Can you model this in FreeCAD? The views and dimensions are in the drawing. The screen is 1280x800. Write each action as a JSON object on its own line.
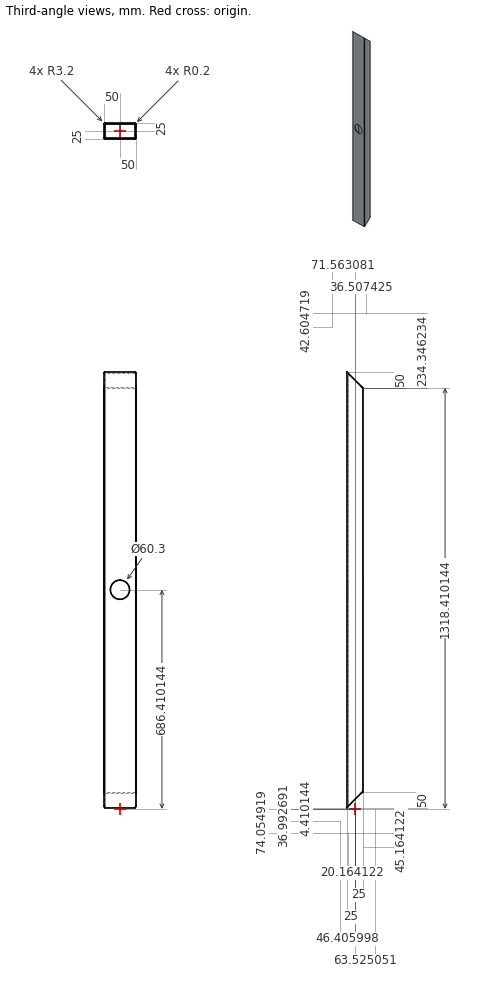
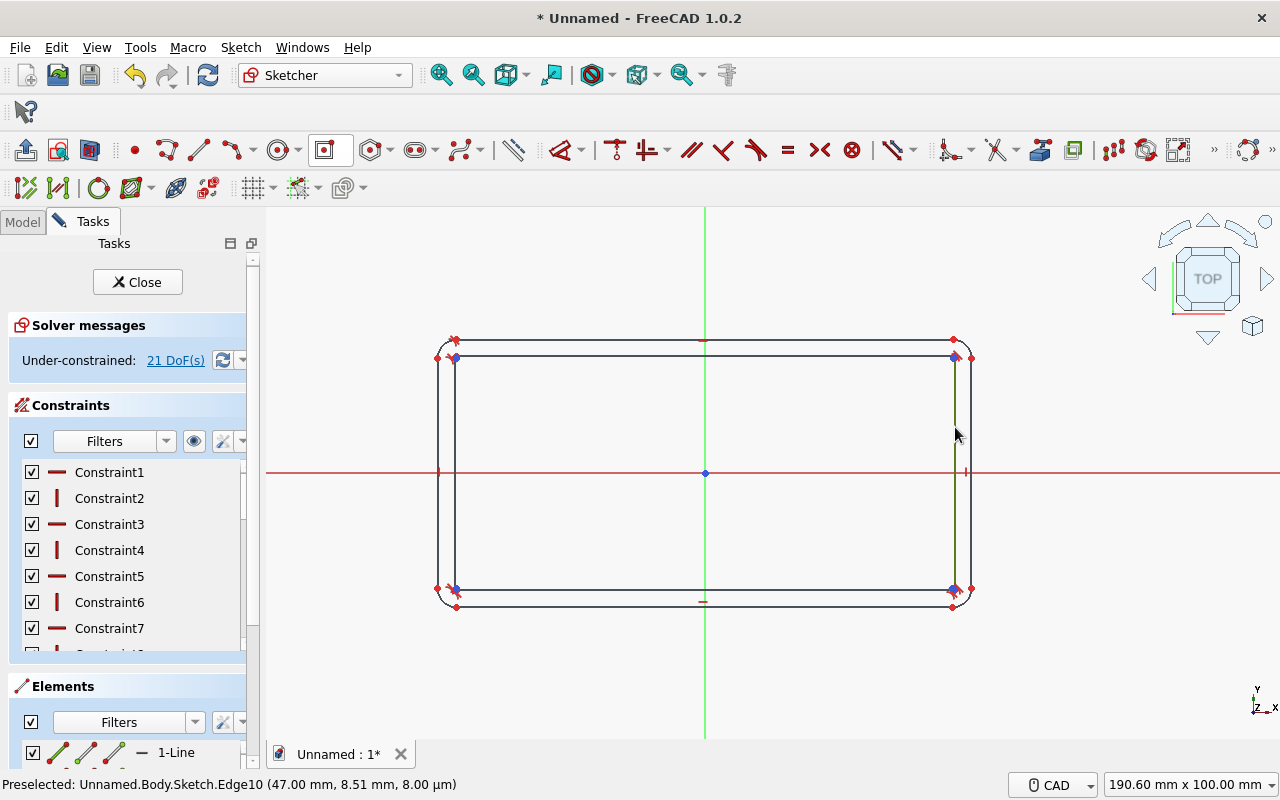
{"action": "scroll", "coordinate": [955, 590], "scroll_direction": "up", "scroll_amount": 14}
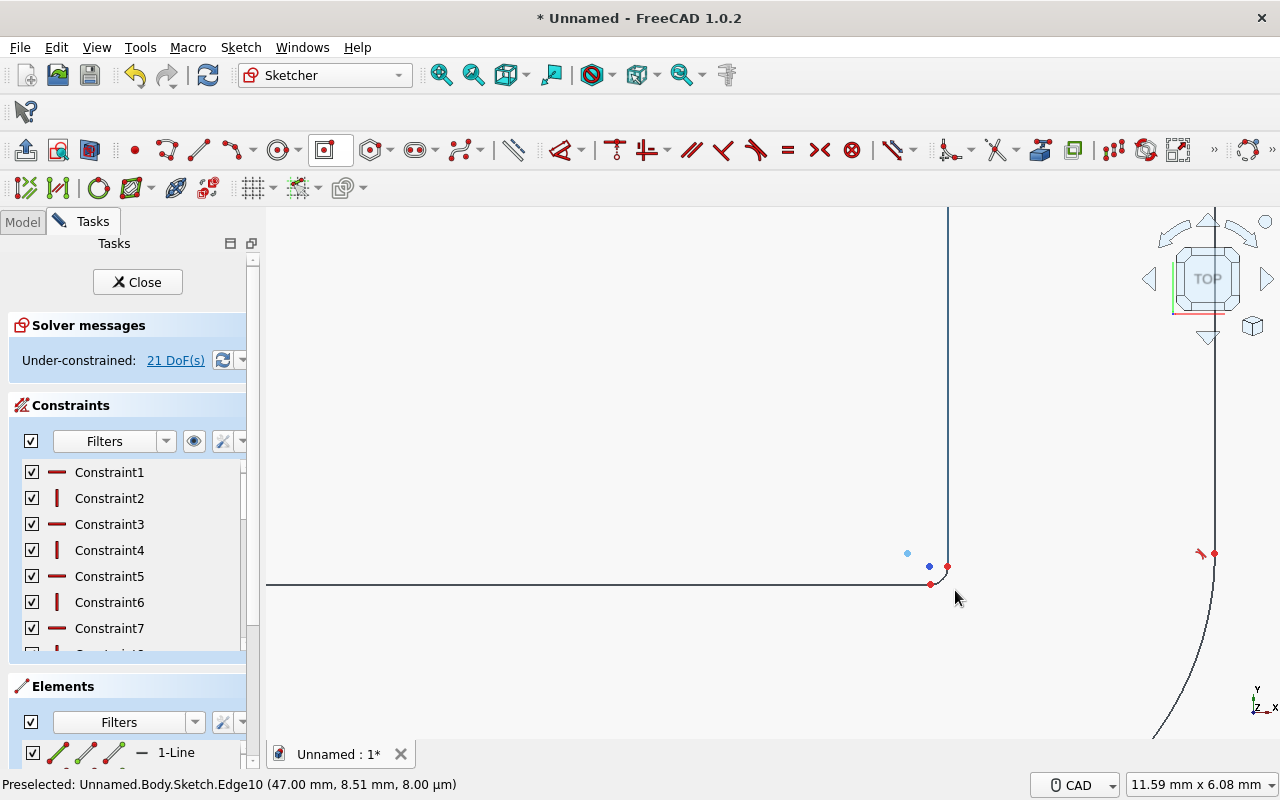
{"action": "left_click", "coordinate": [943, 579]}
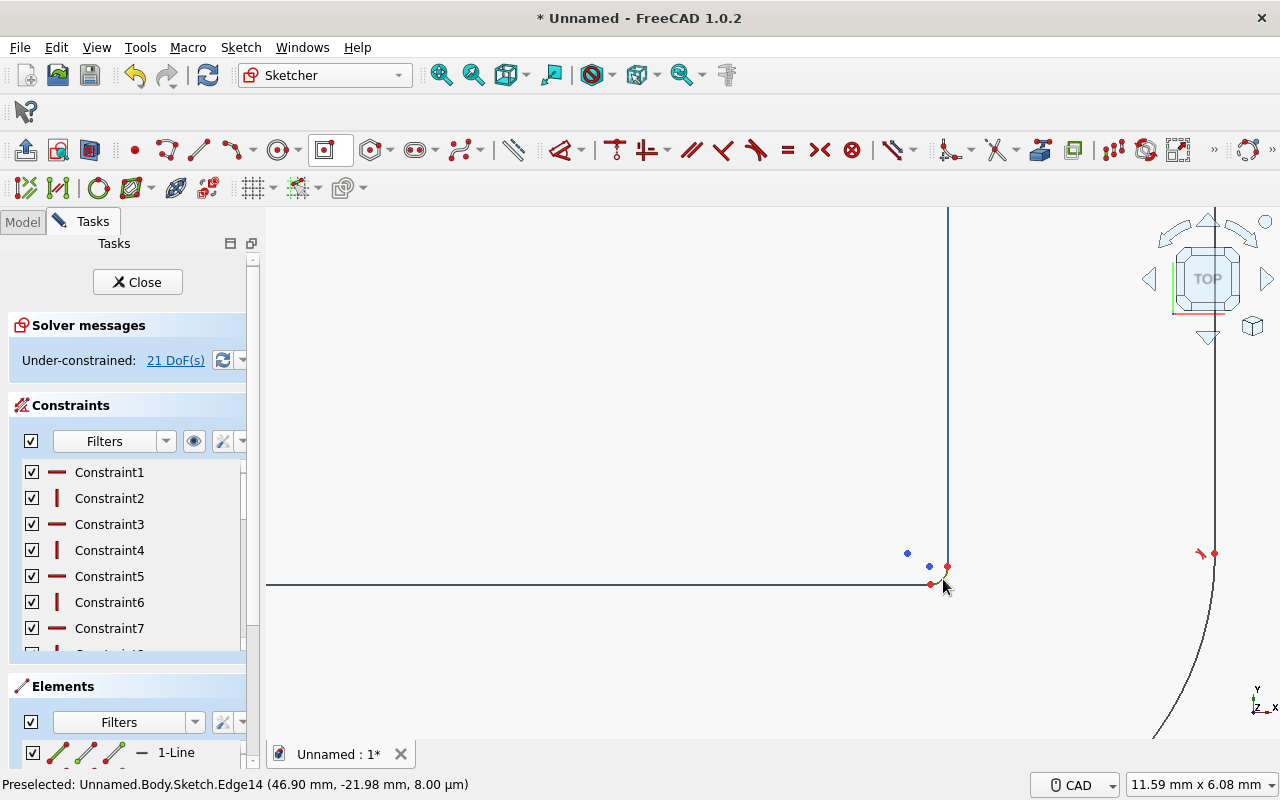
{"action": "key", "text": "t"}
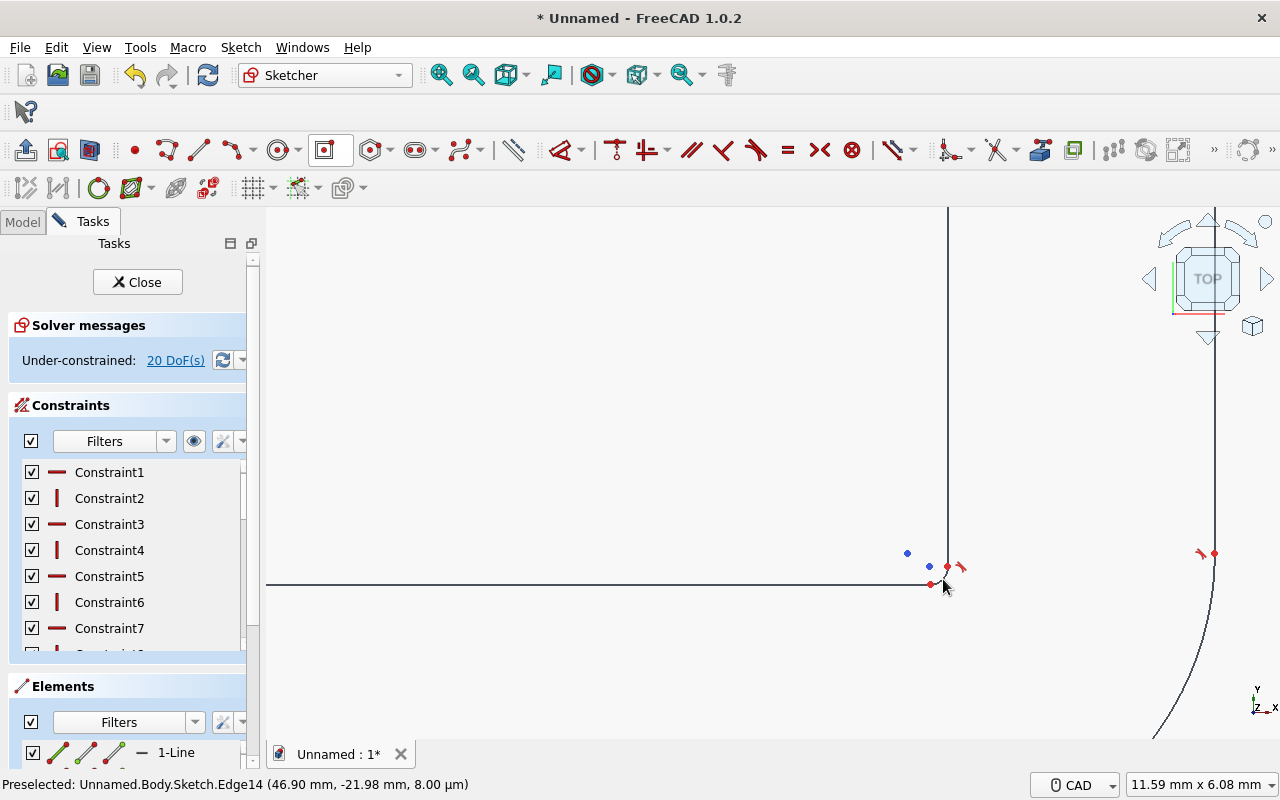
{"action": "scroll", "coordinate": [955, 590], "scroll_direction": "down", "scroll_amount": 14}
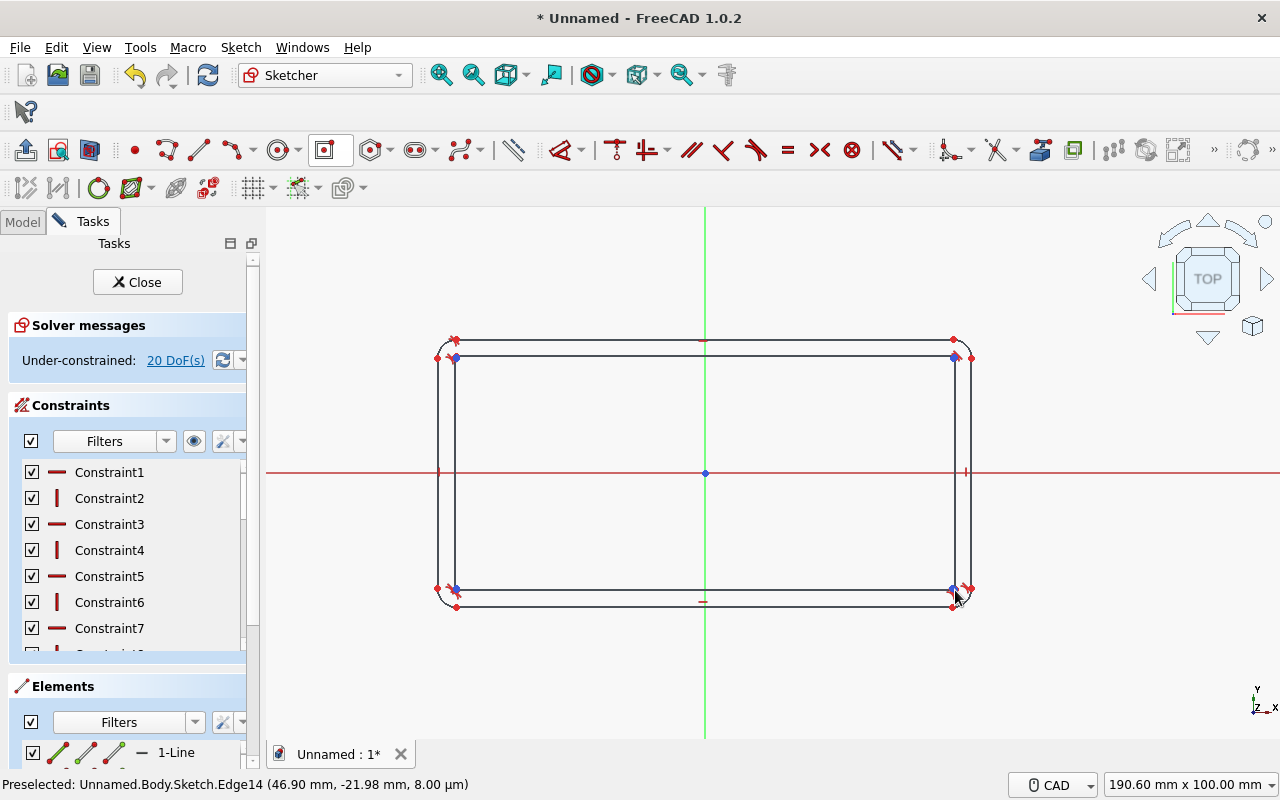
{"action": "left_click", "coordinate": [805, 590]}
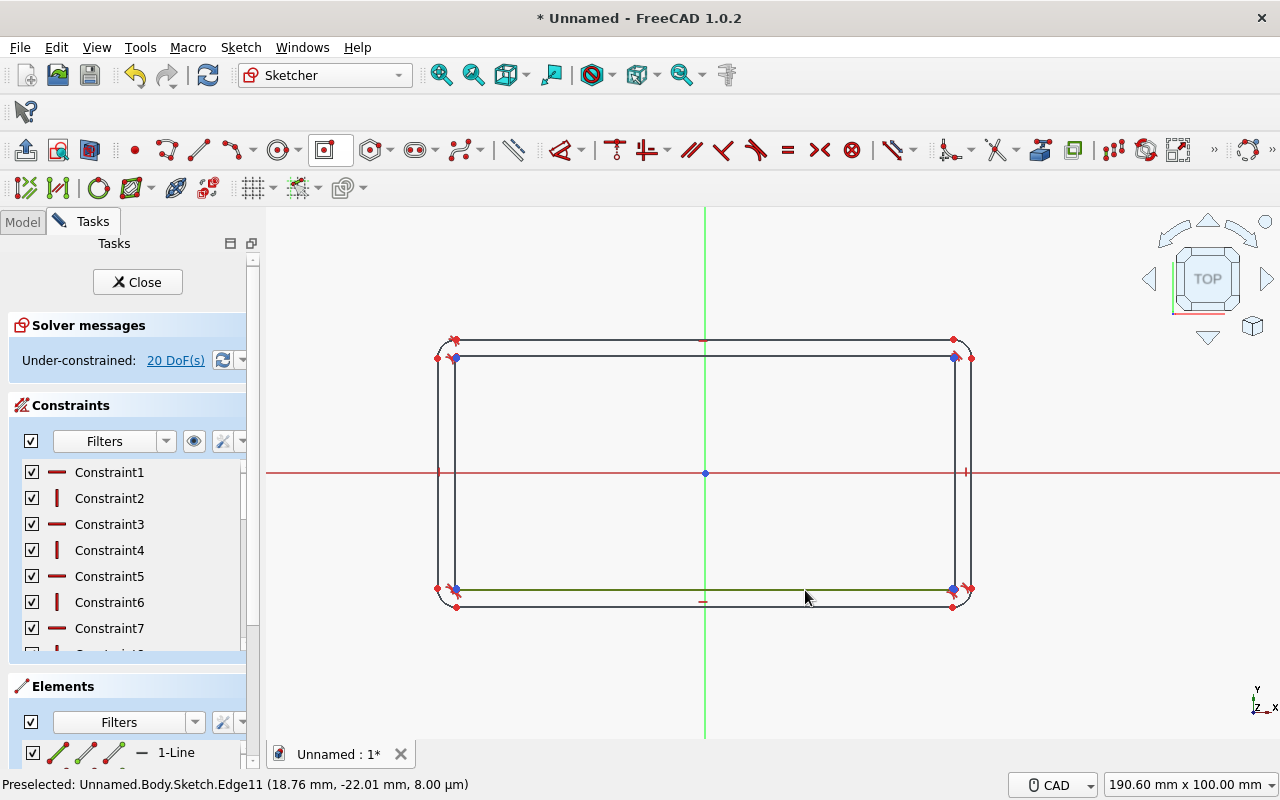
{"action": "scroll", "coordinate": [955, 590], "scroll_direction": "up", "scroll_amount": 14}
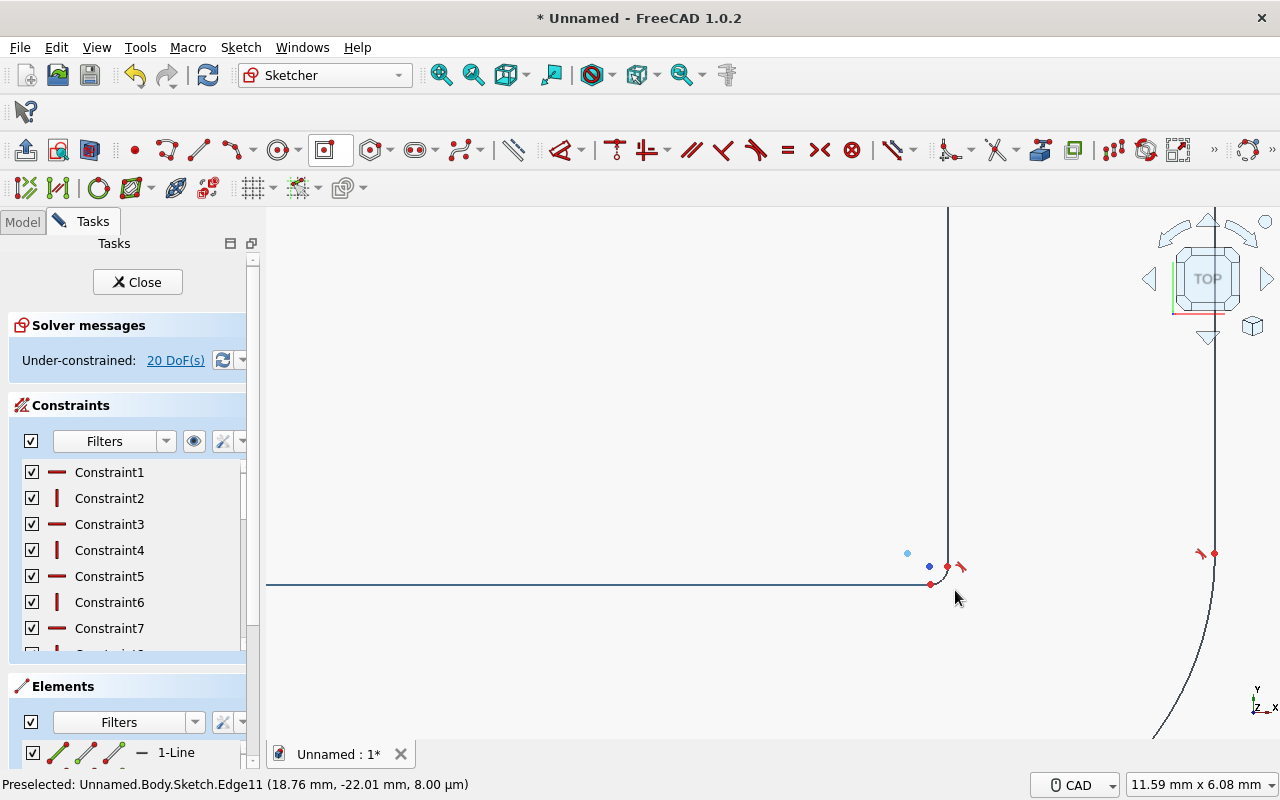
{"action": "left_click", "coordinate": [943, 579]}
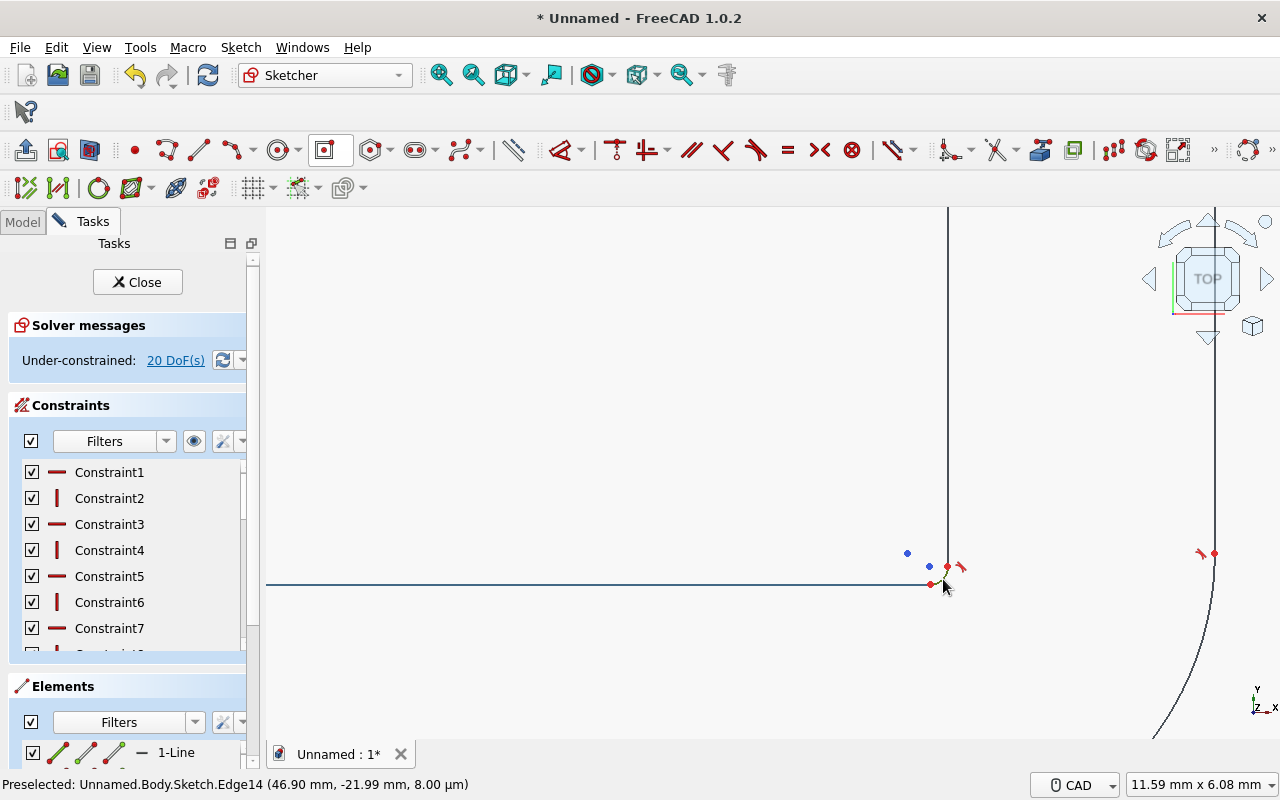
{"action": "left_click", "coordinate": [756, 150]}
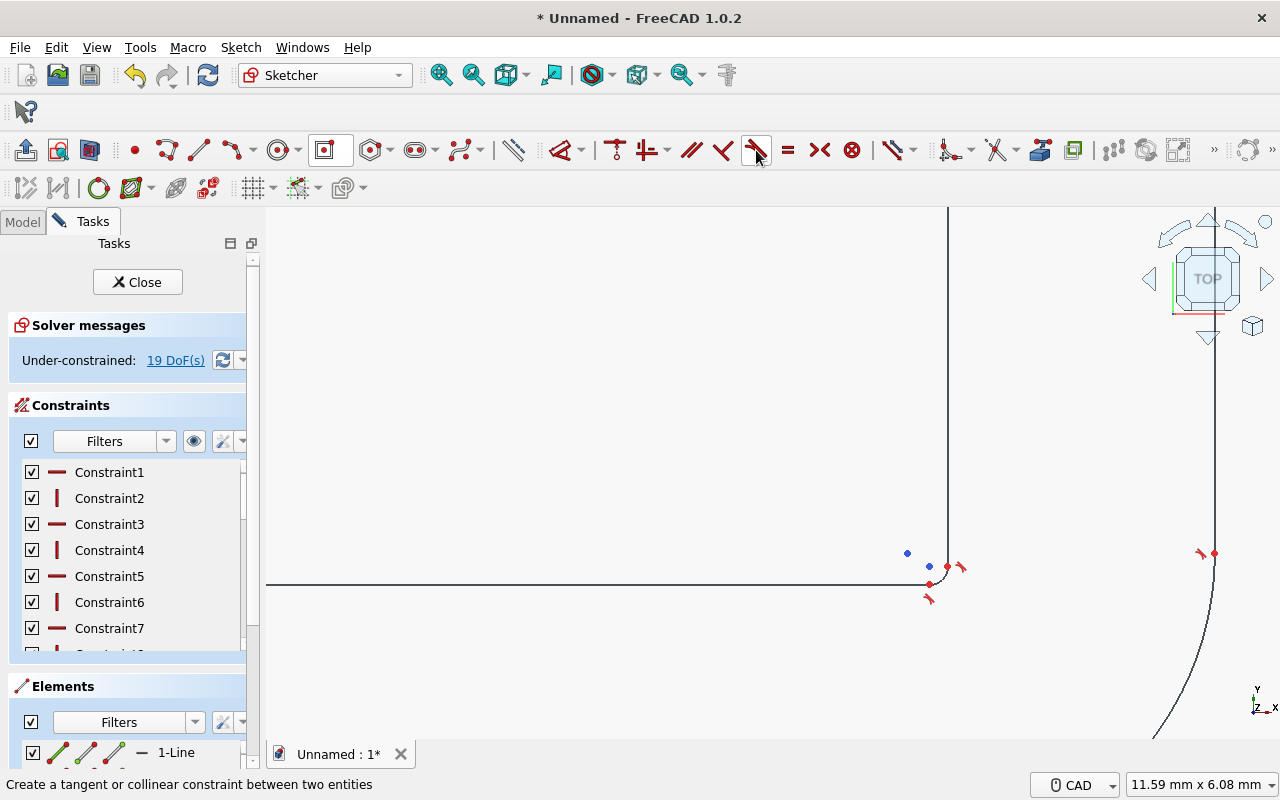
{"action": "scroll", "coordinate": [955, 590], "scroll_direction": "down", "scroll_amount": 14}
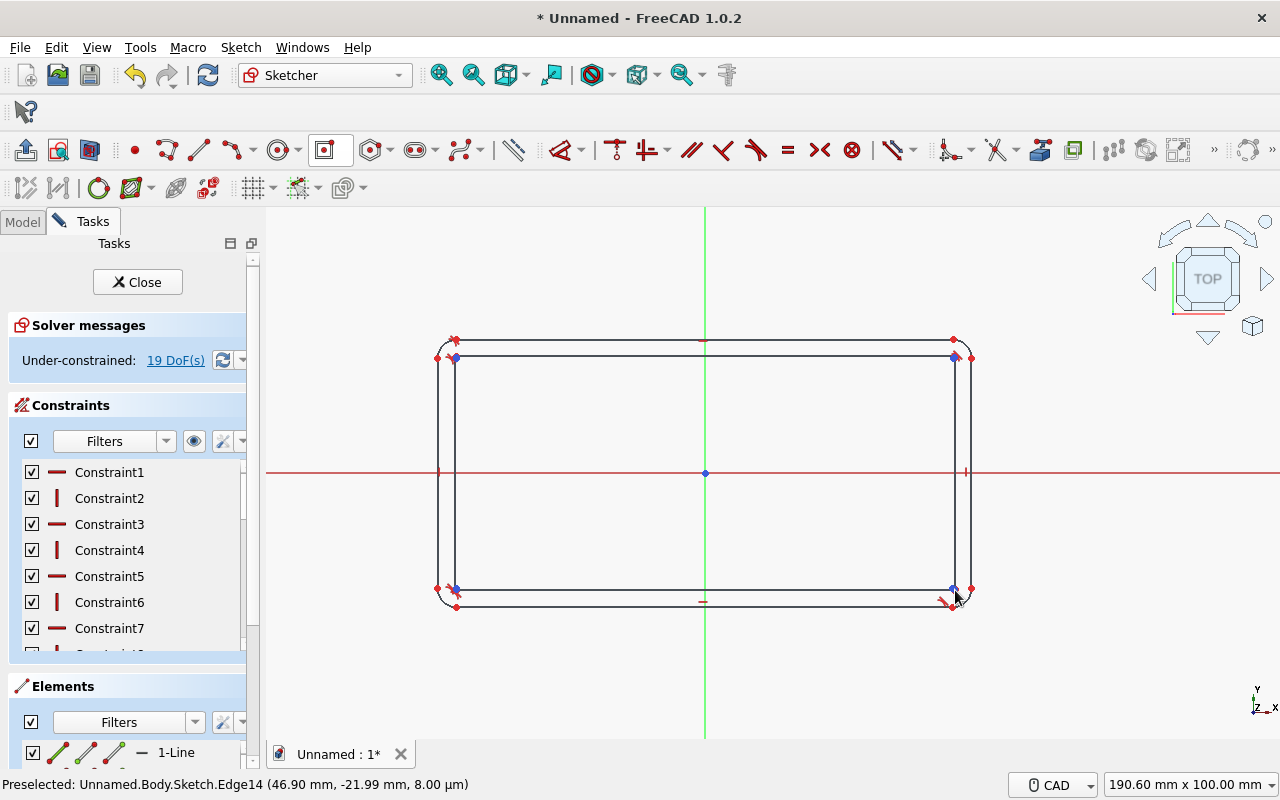
{"action": "left_click", "coordinate": [805, 590]}